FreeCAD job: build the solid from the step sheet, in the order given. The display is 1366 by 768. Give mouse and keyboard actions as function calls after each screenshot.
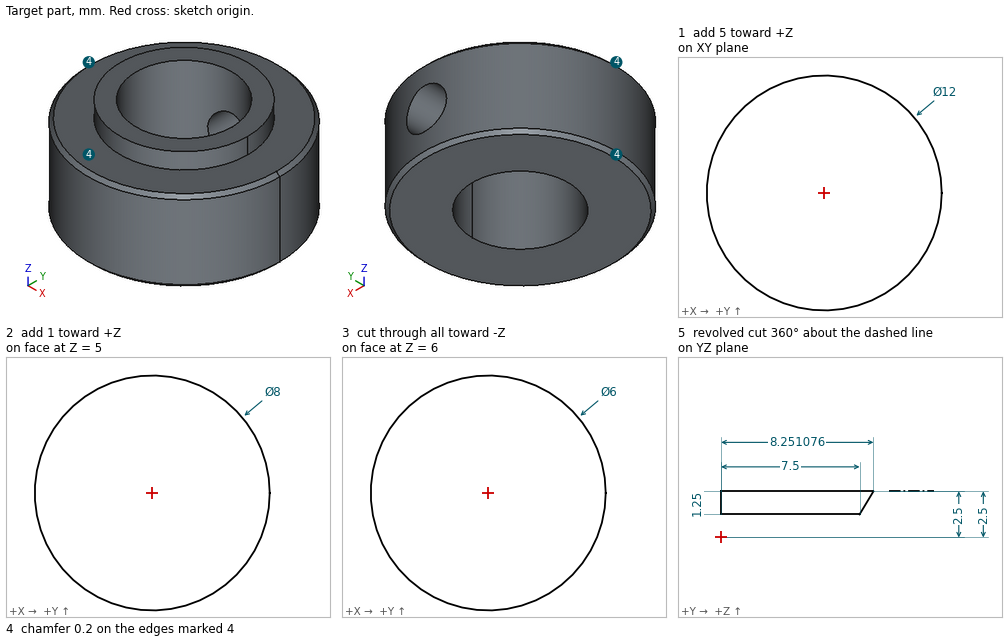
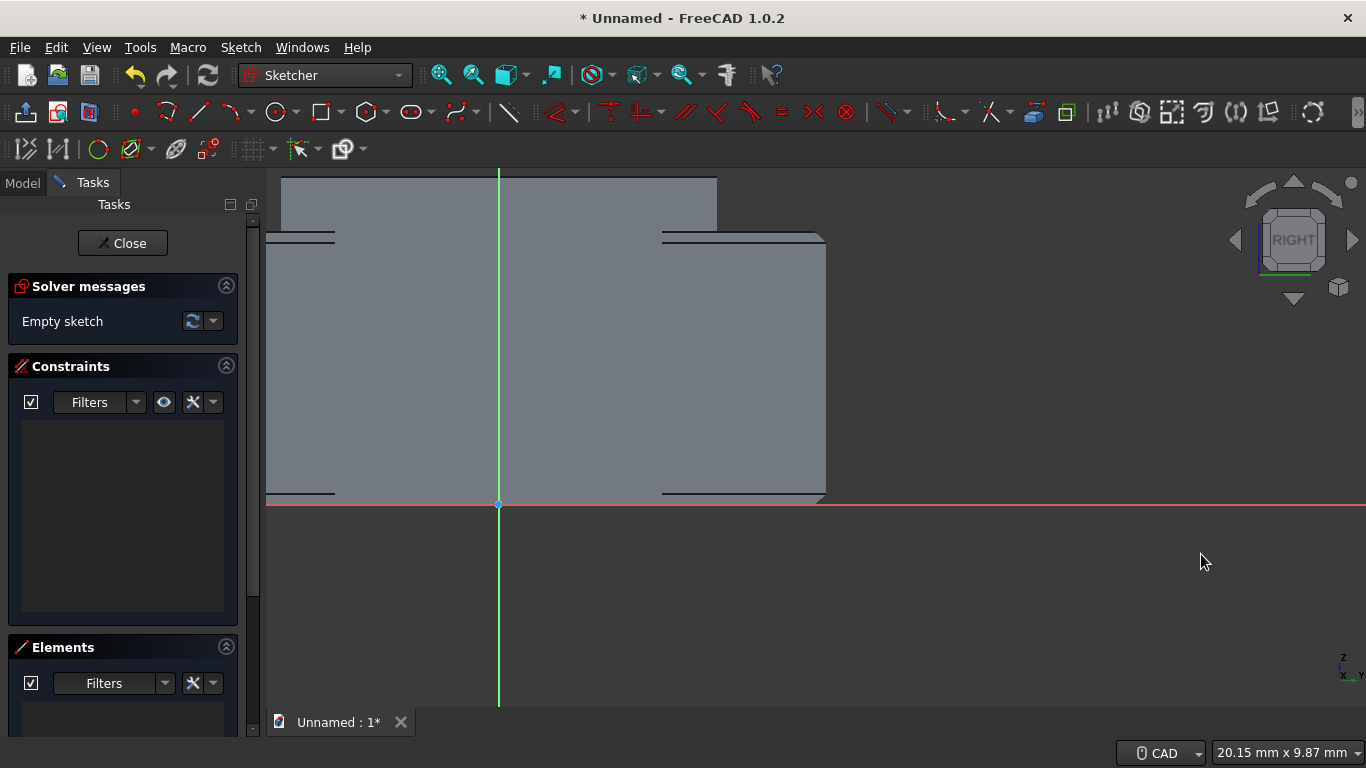
click(168, 112)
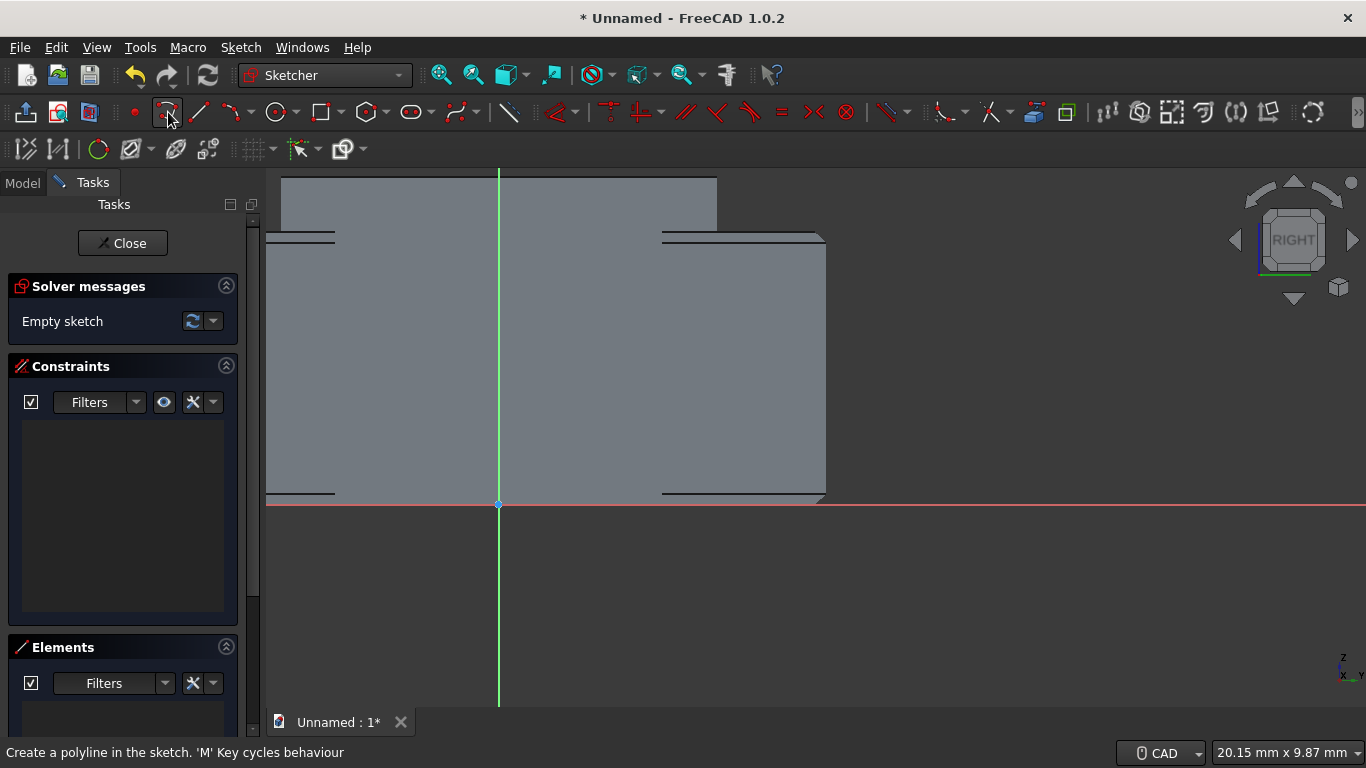
click(499, 437)
click(908, 437)
click(949, 368)
click(508, 368)
click(499, 438)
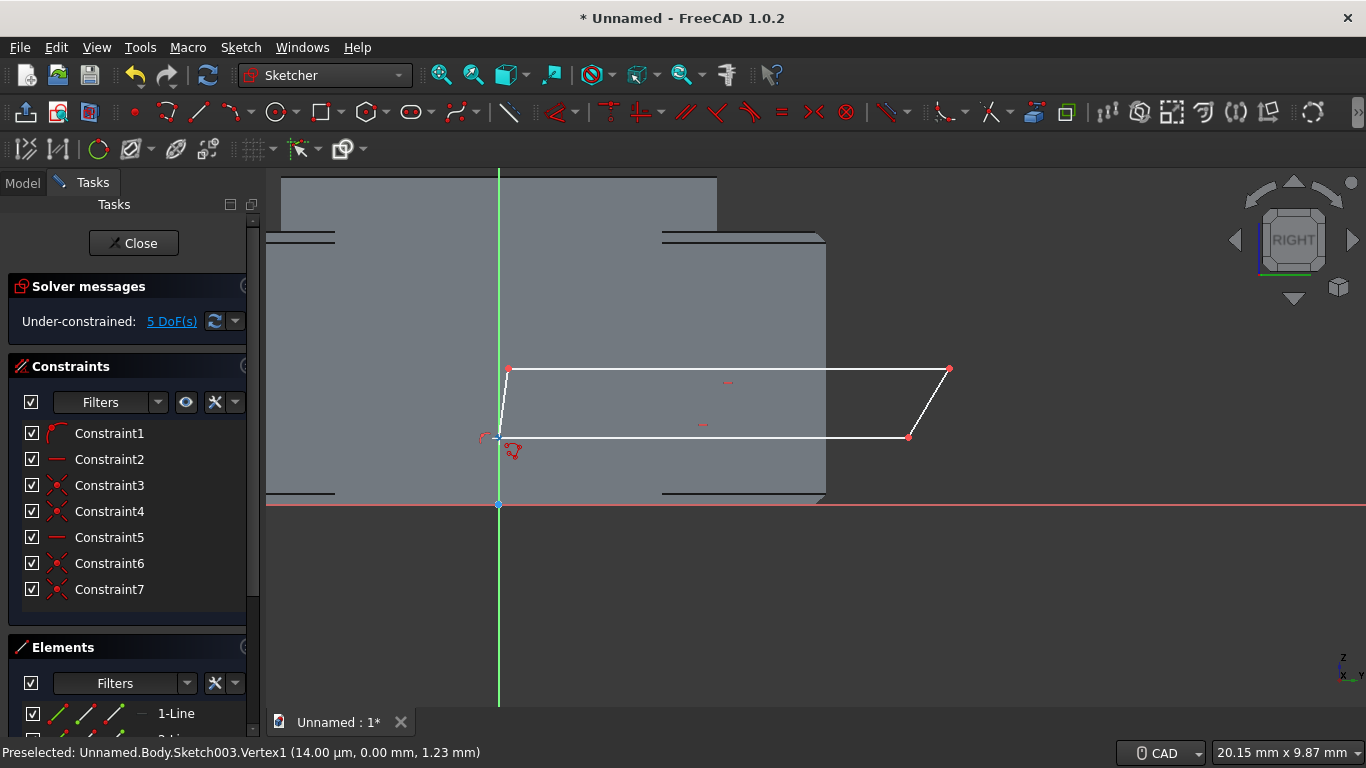
key(g)
key(l)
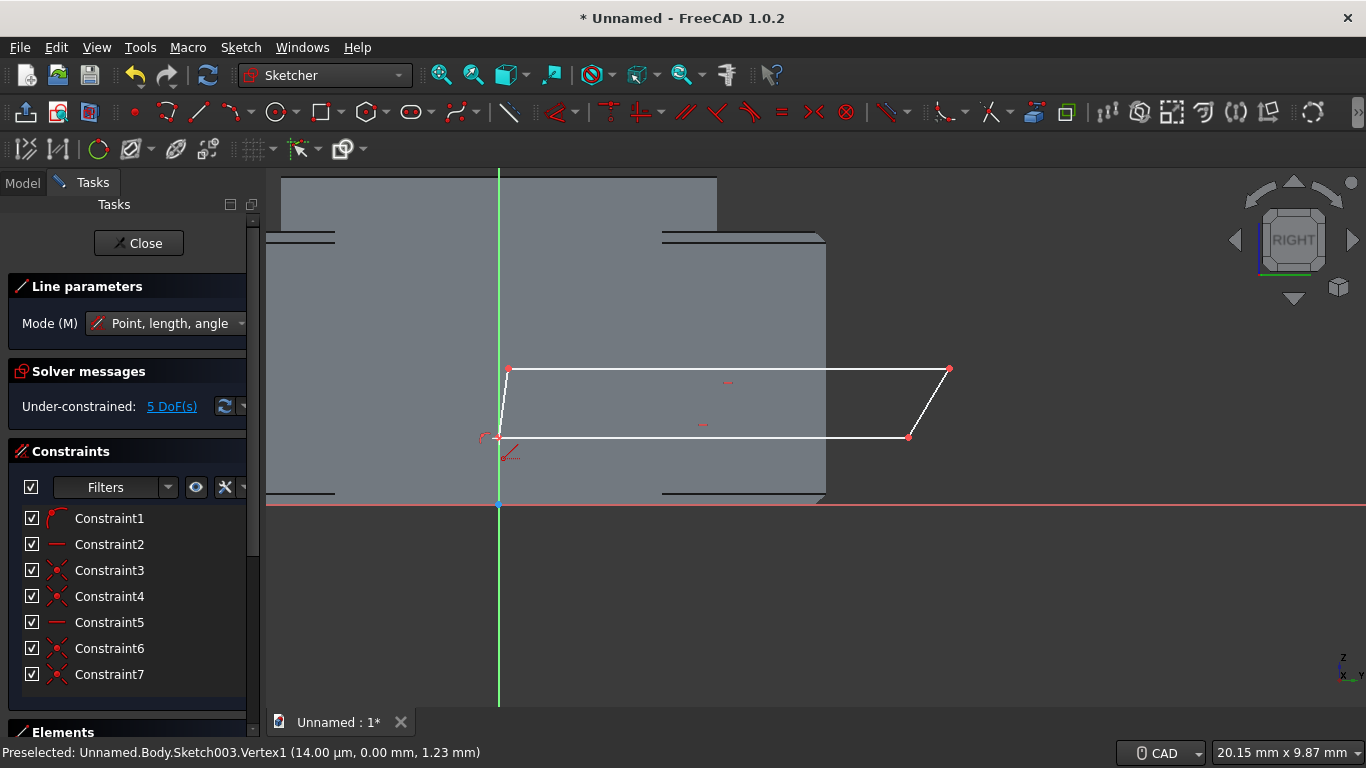
click(994, 368)
click(1129, 368)
key(Escape)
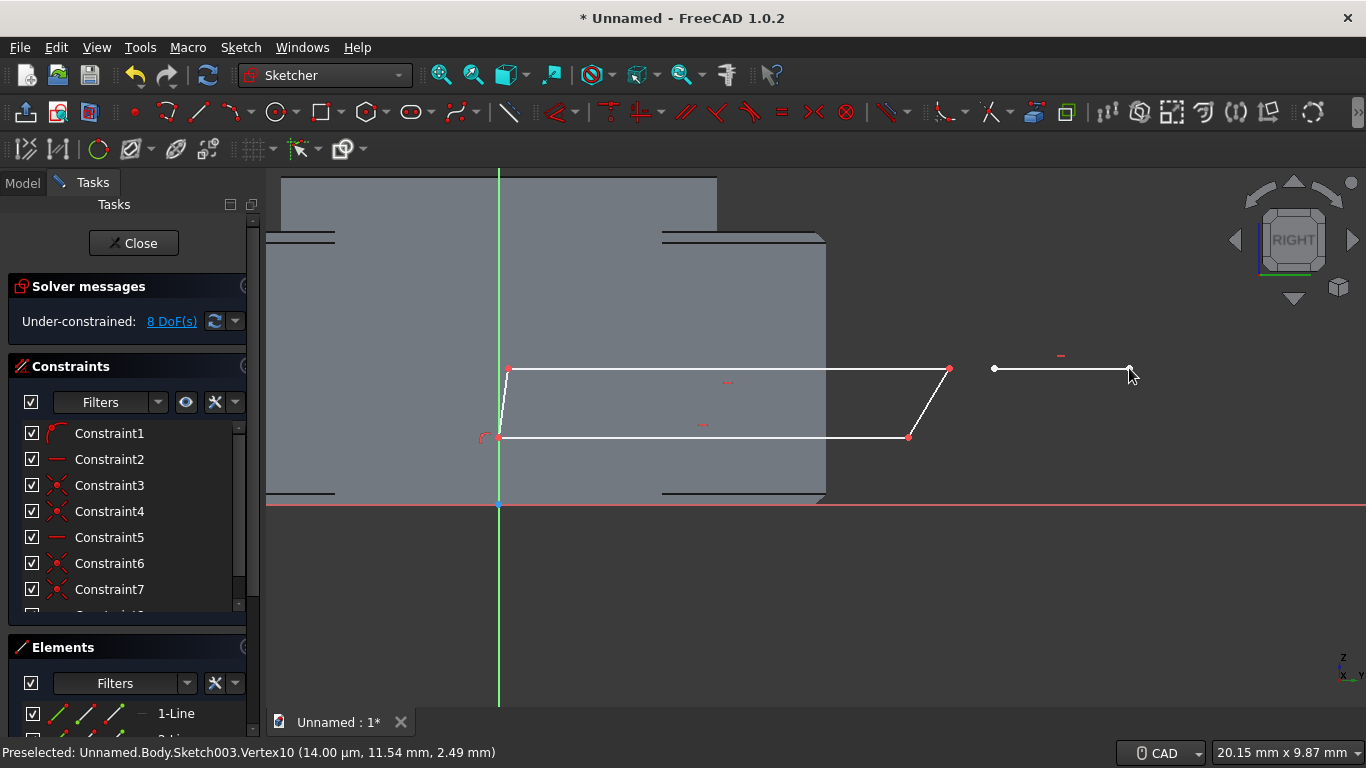
click(1034, 369)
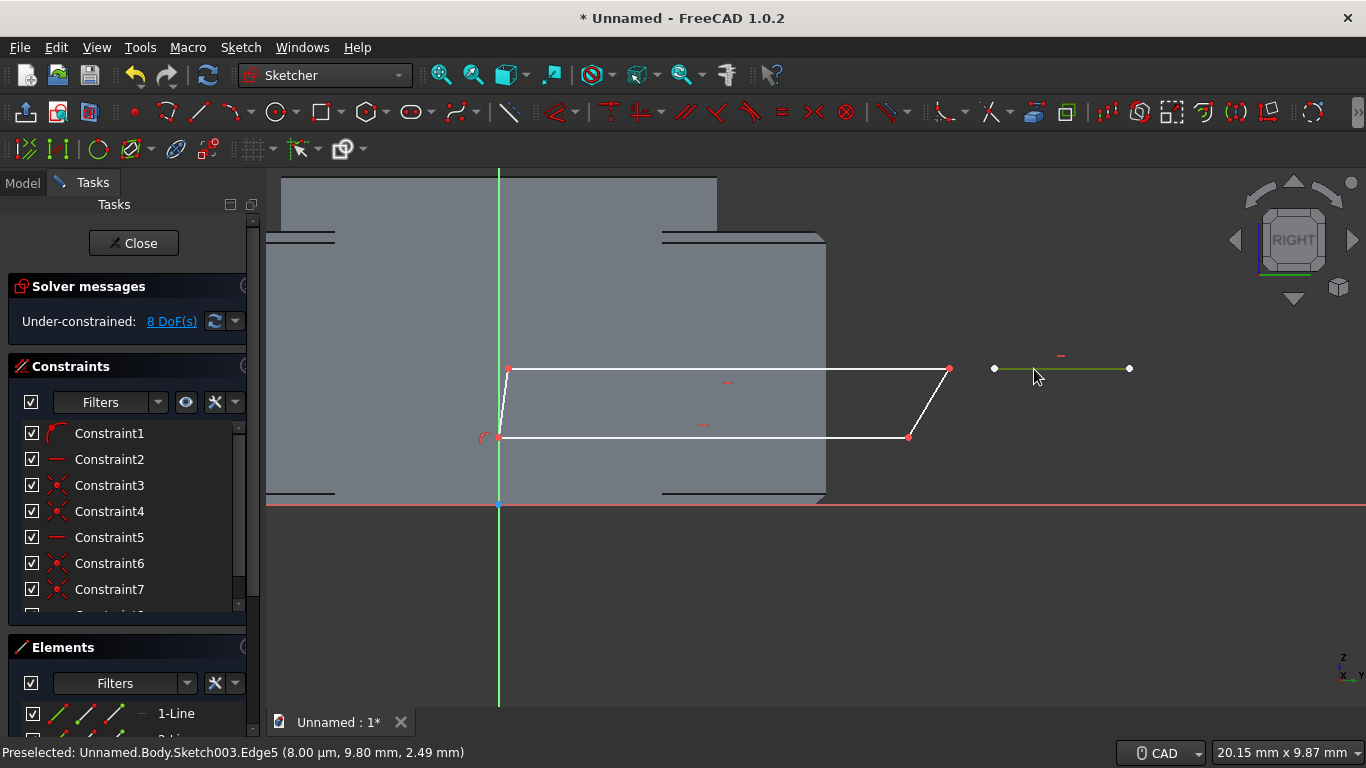
click(510, 112)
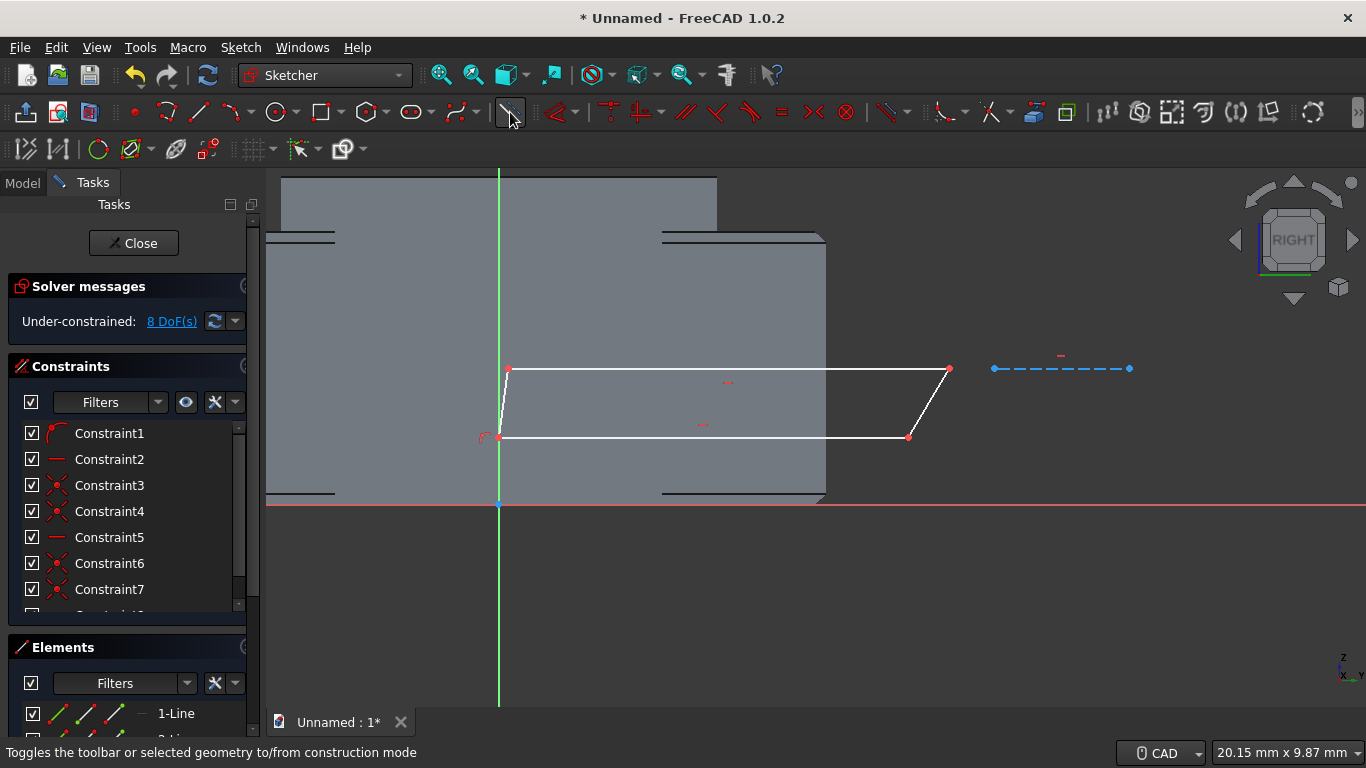
click(502, 417)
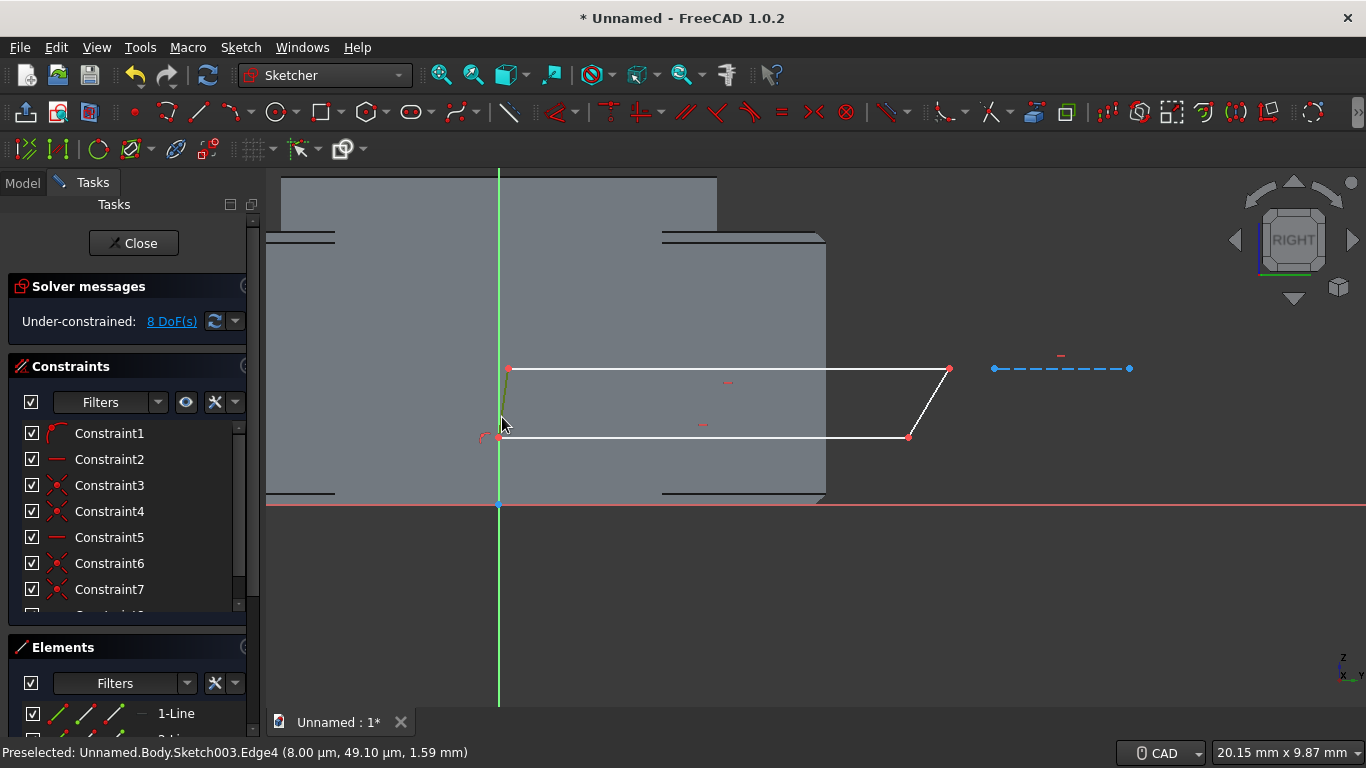
click(664, 112)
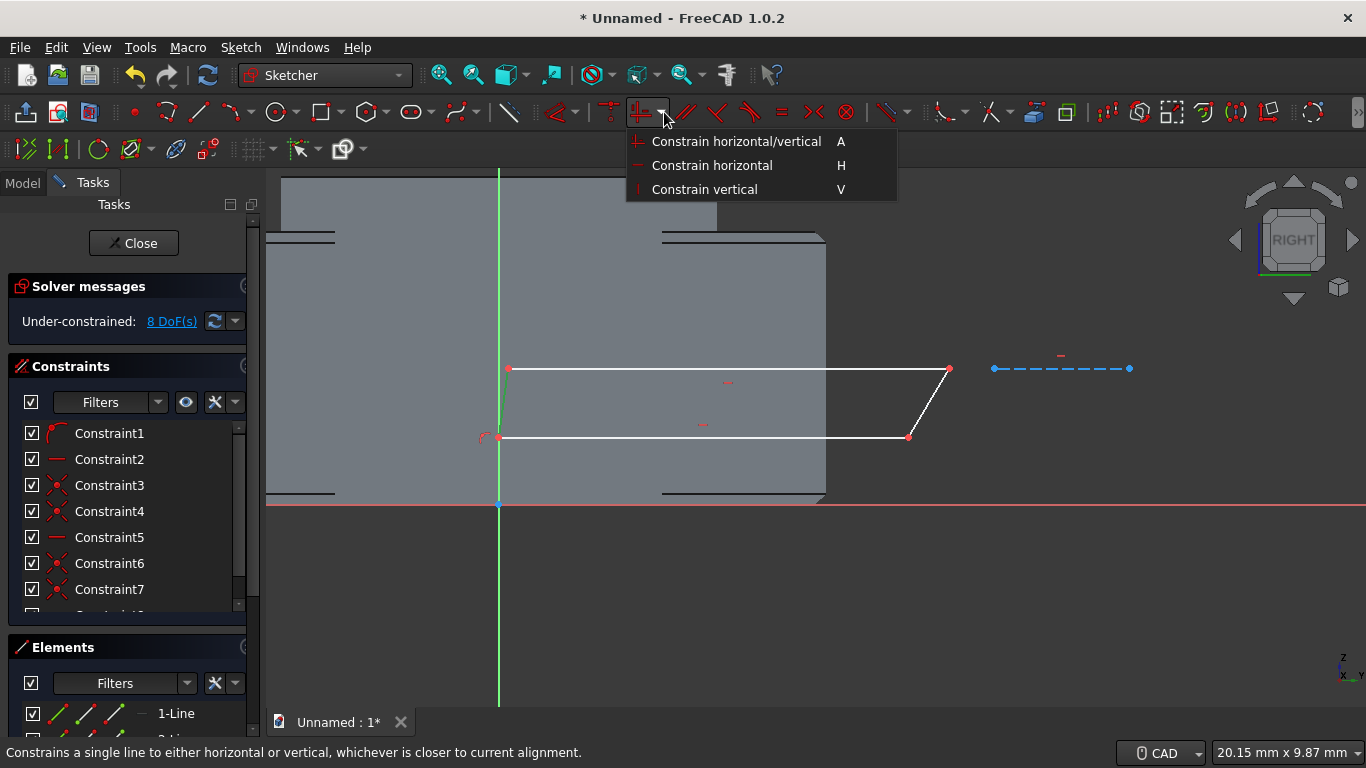
click(762, 189)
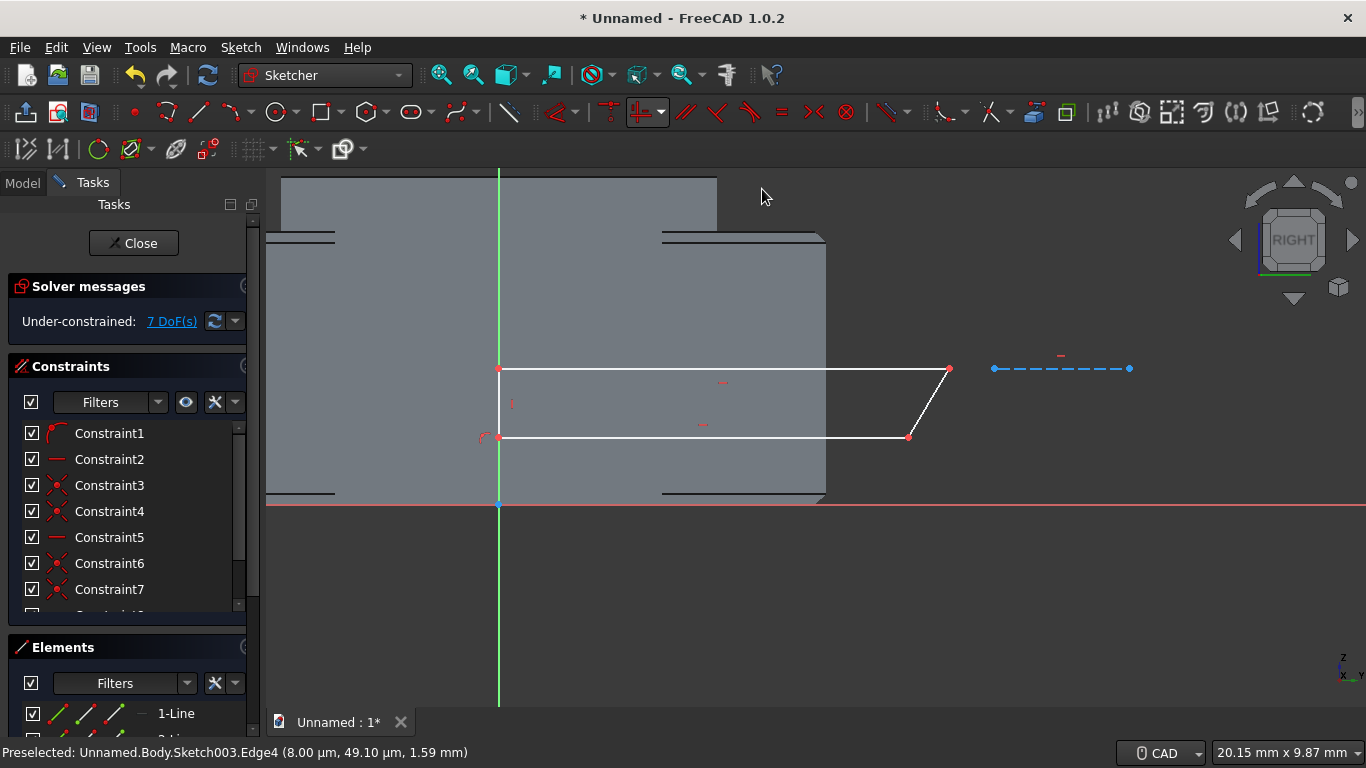
click(556, 112)